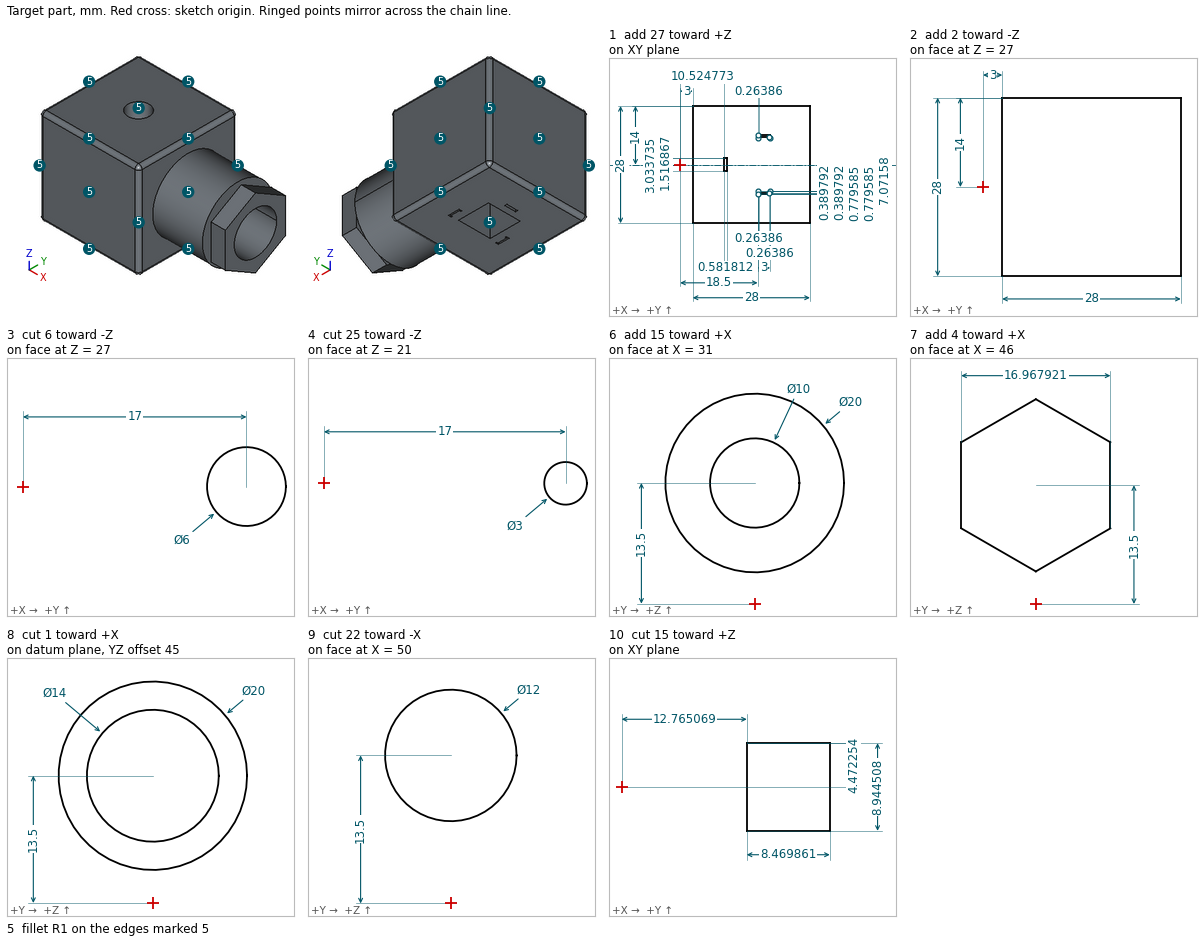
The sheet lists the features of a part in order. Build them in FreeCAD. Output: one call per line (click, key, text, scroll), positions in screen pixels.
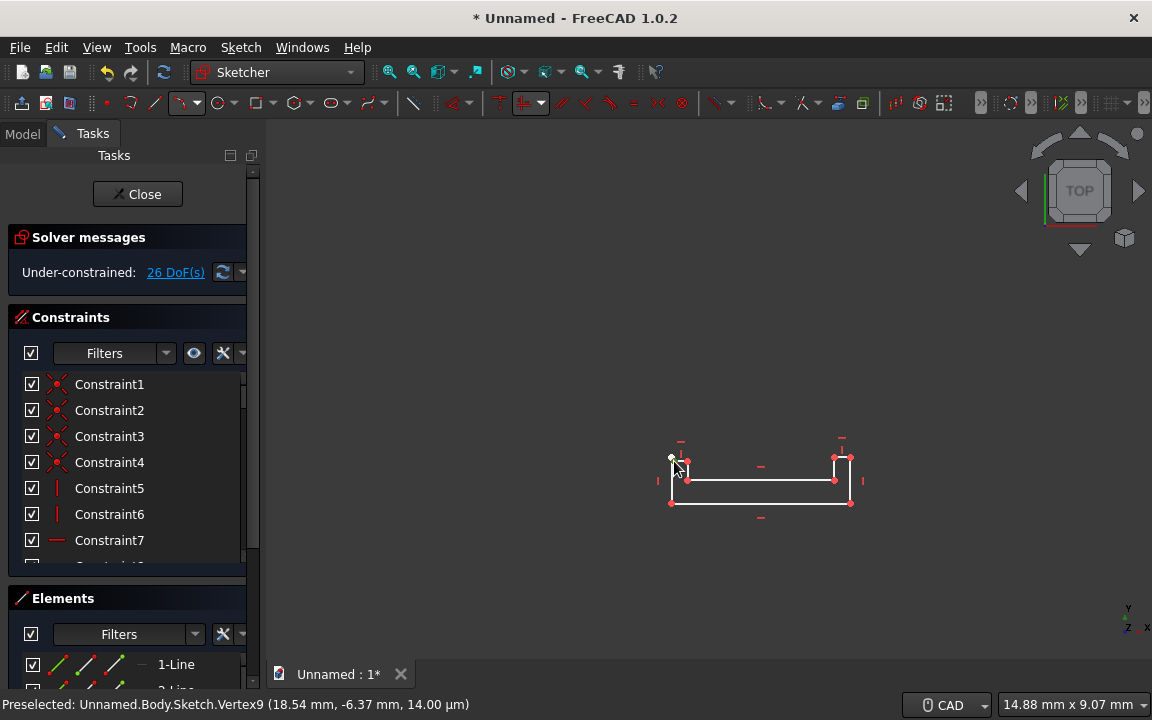
scroll(678, 467, down, 8)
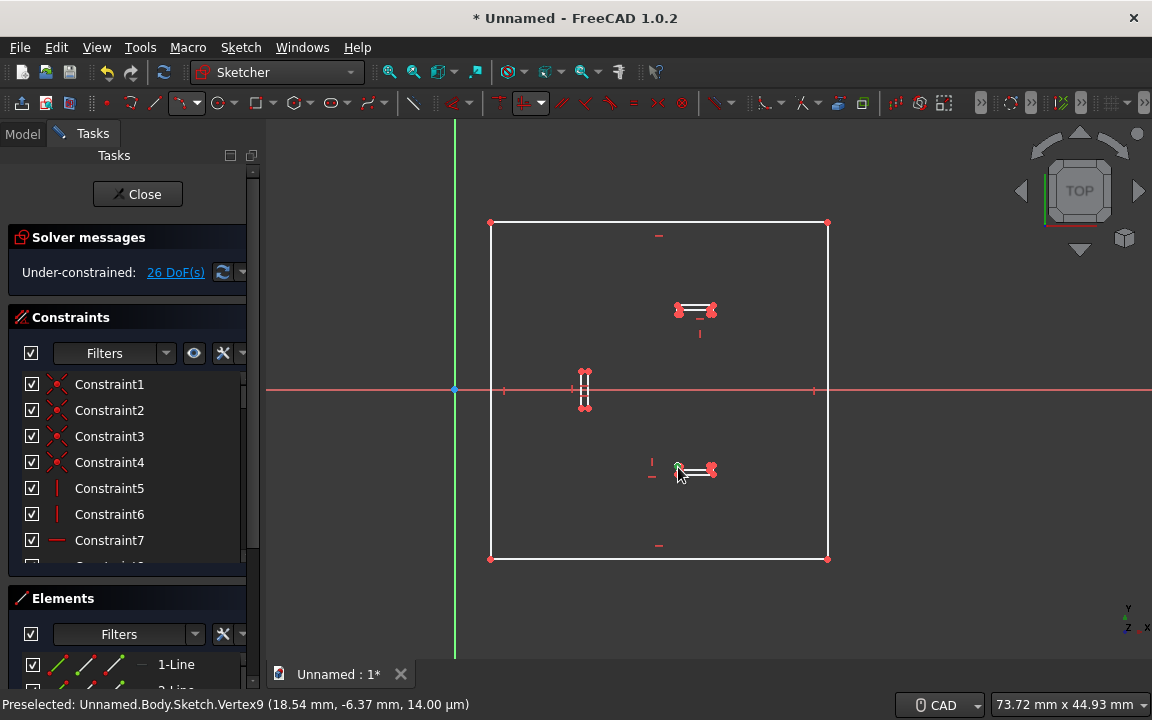
scroll(677, 314, up, 8)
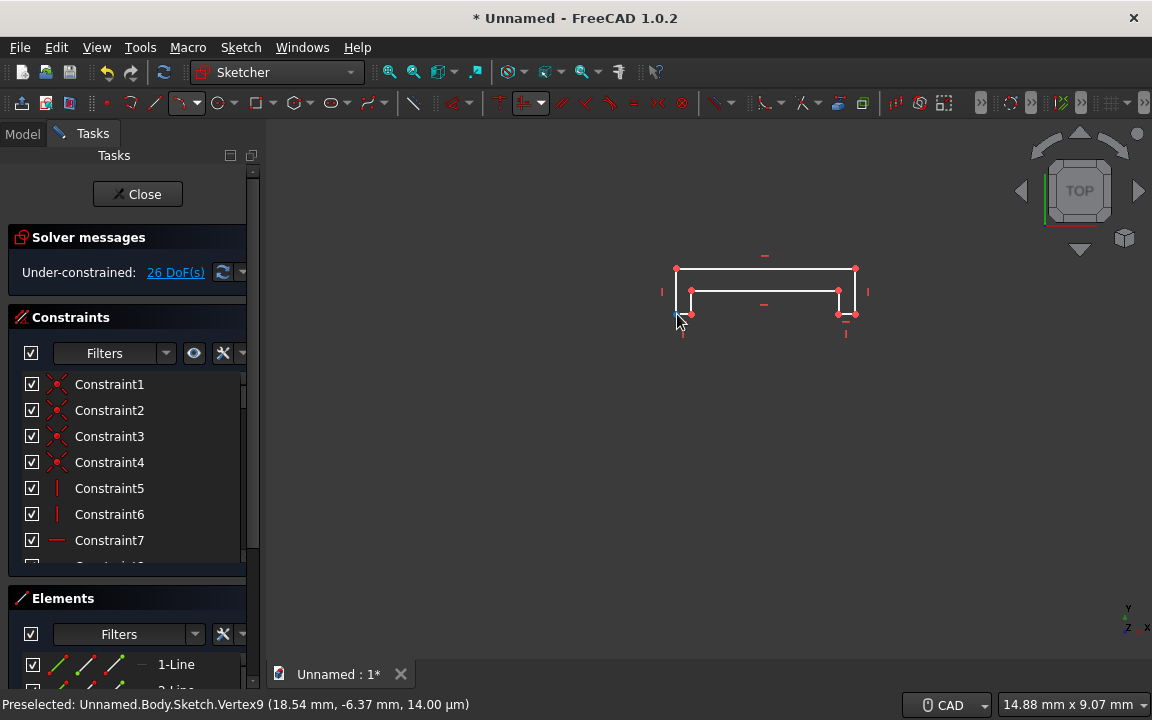
click(676, 314)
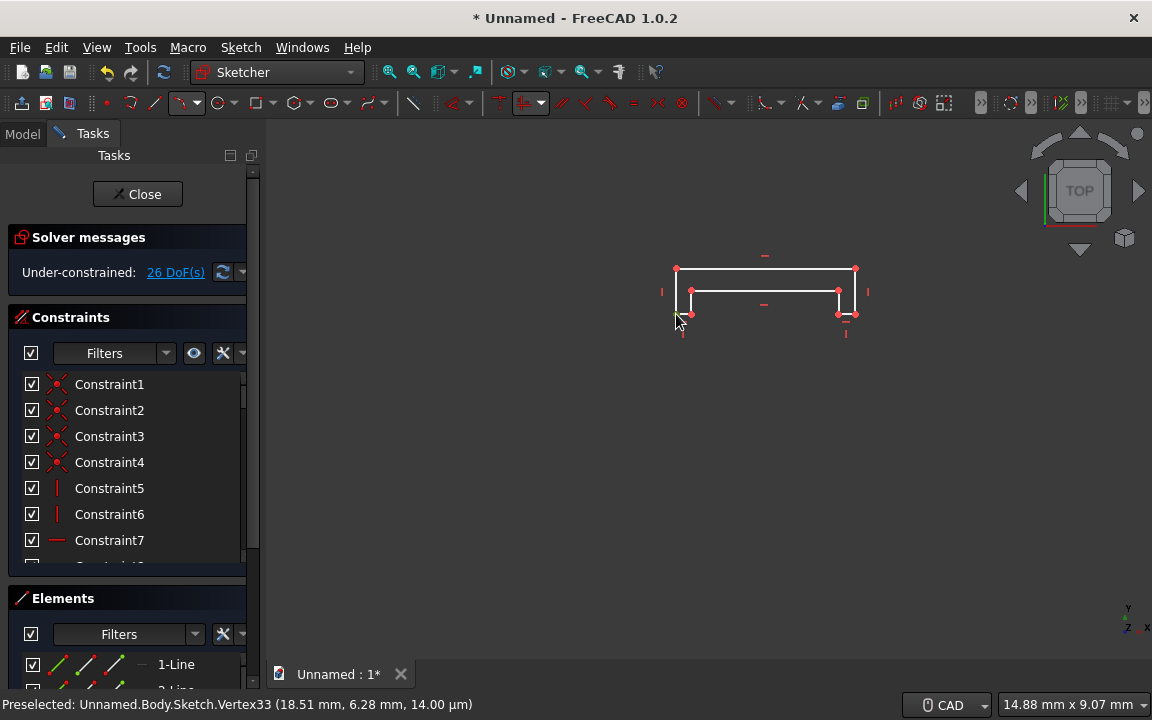
scroll(677, 313, down, 8)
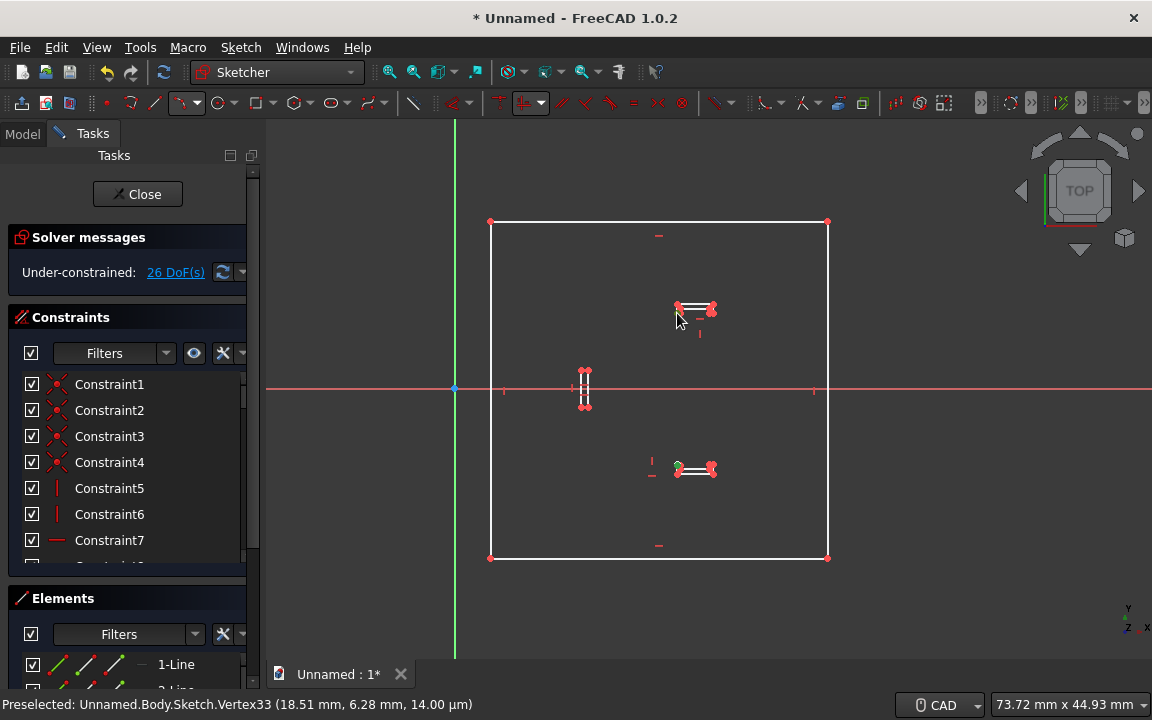
click(344, 389)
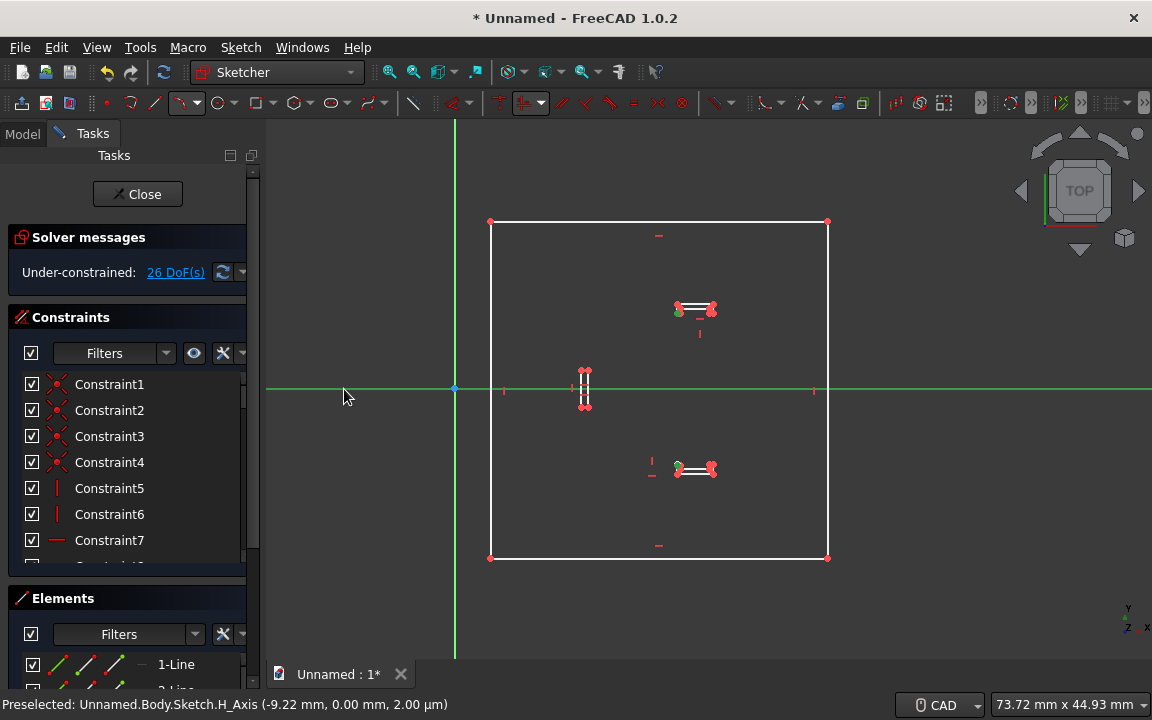
click(658, 104)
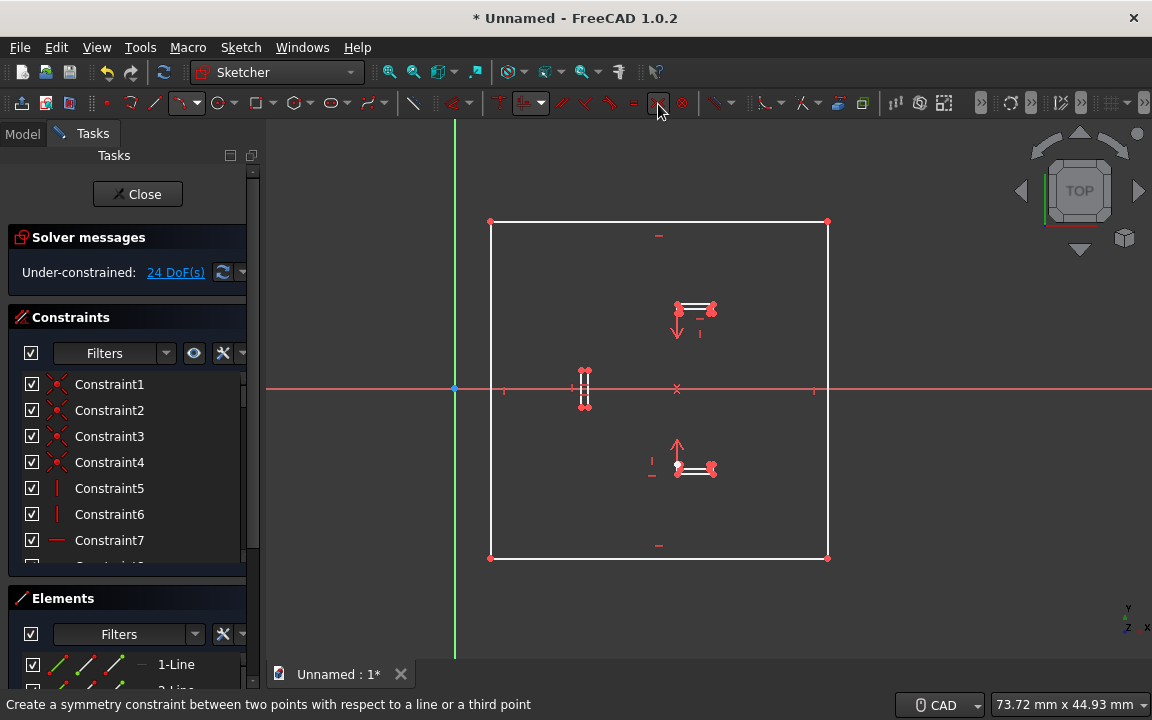
scroll(677, 474, up, 4)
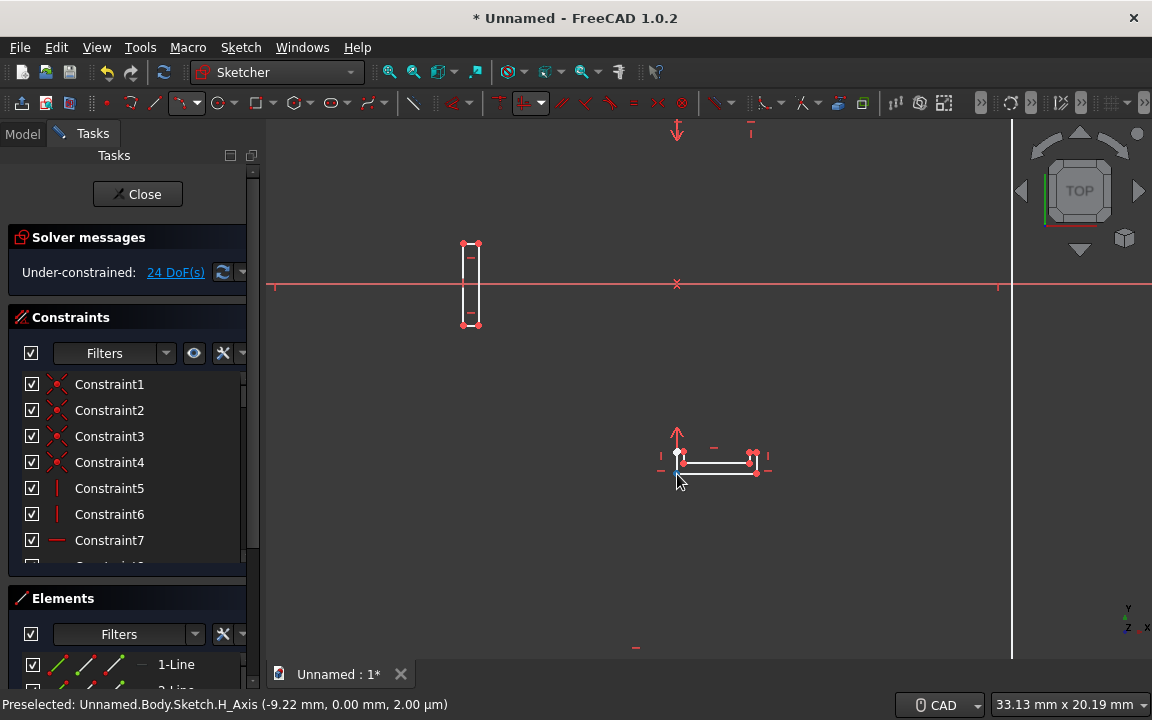
click(677, 474)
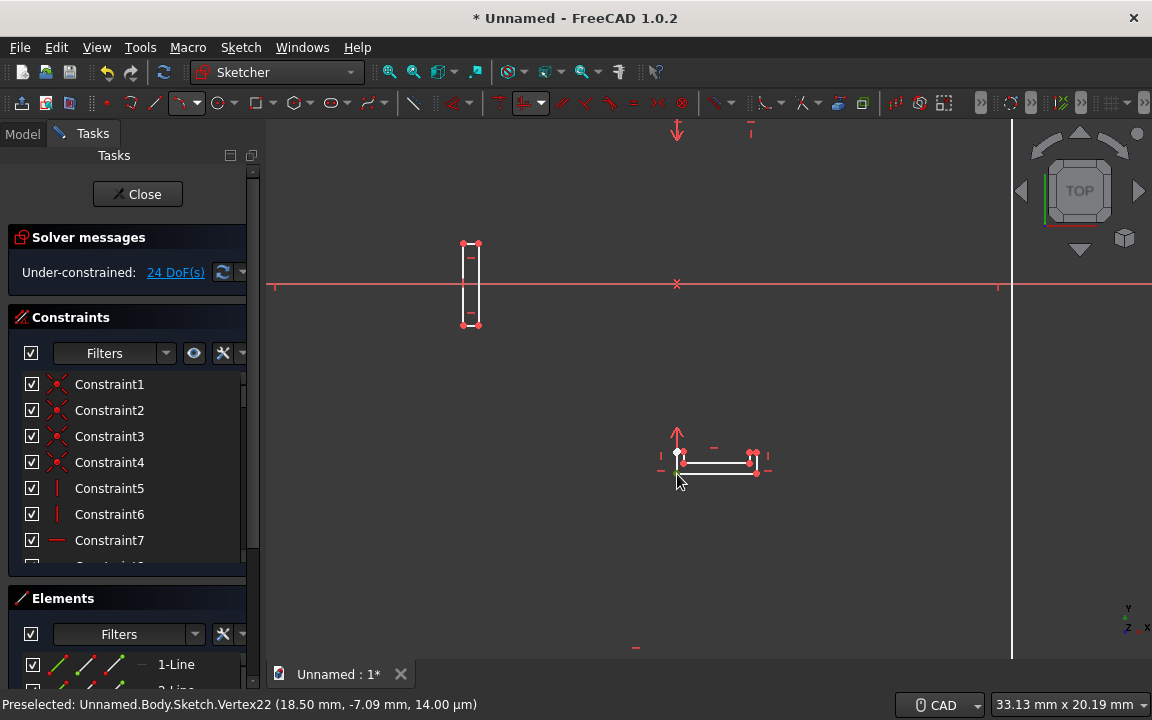
scroll(676, 475, down, 4)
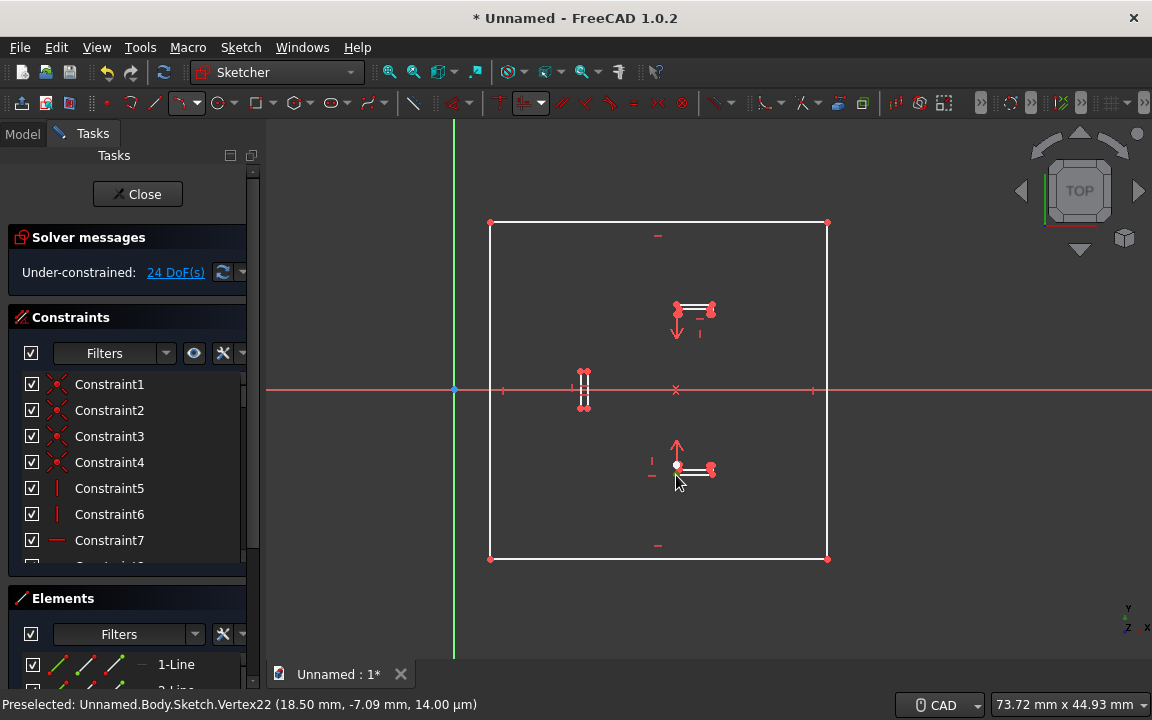
scroll(677, 305, up, 5)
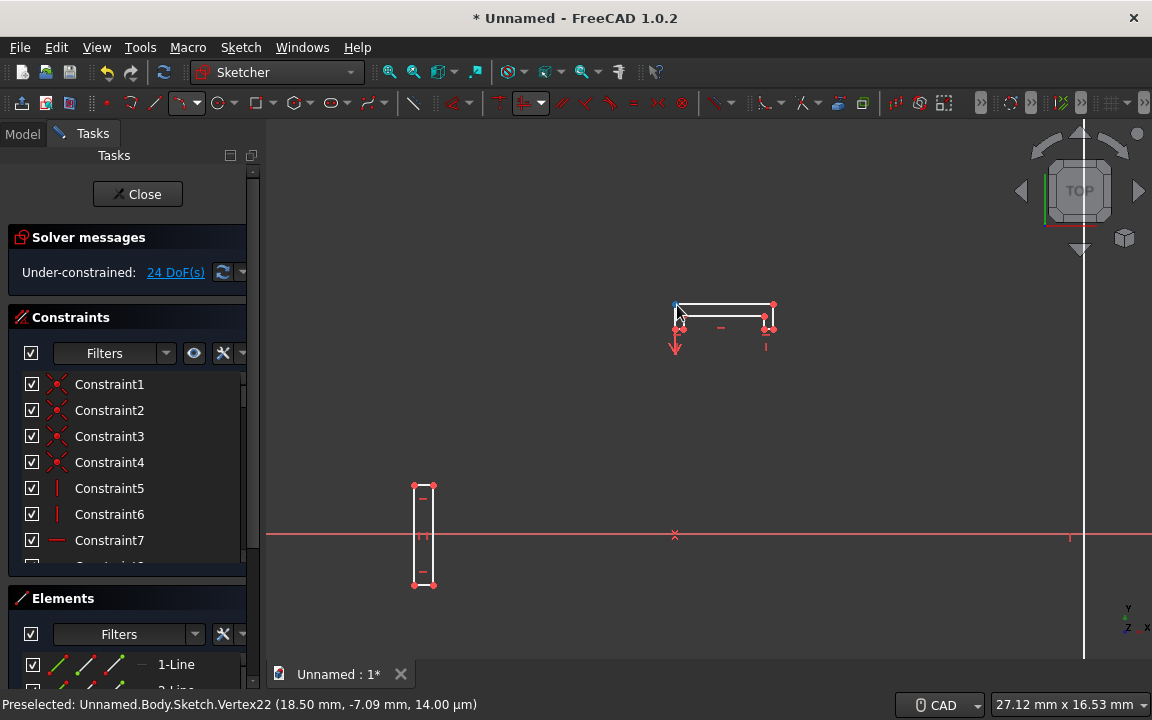
click(675, 304)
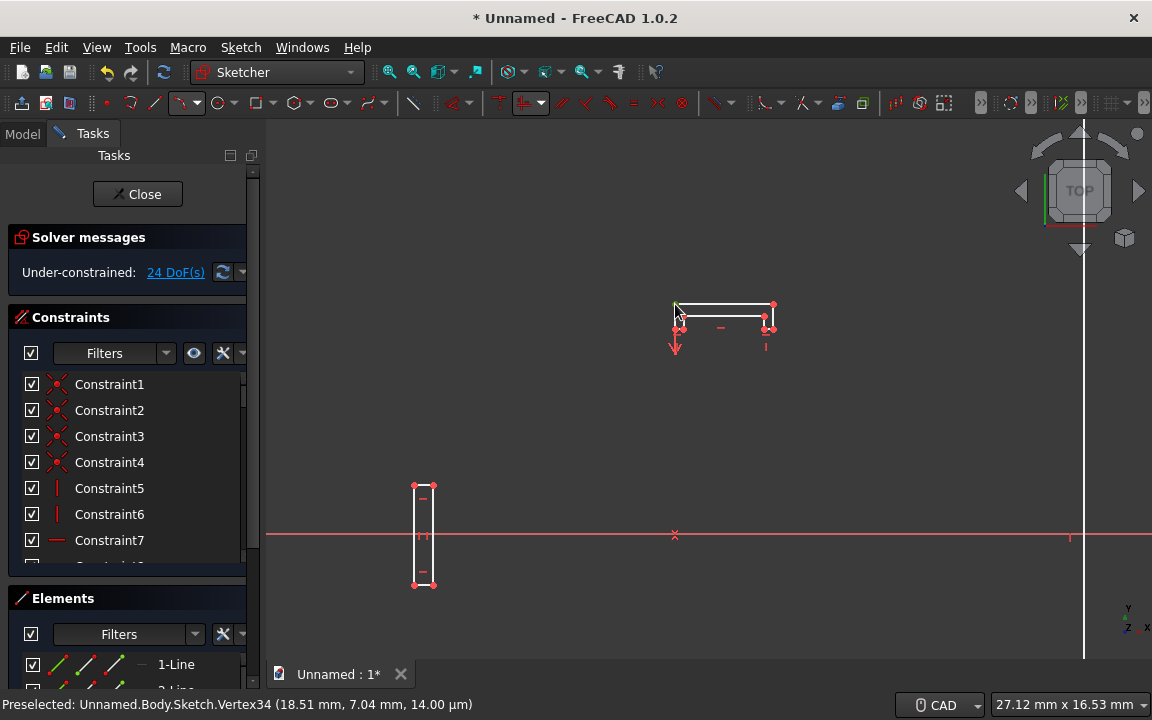
click(344, 534)